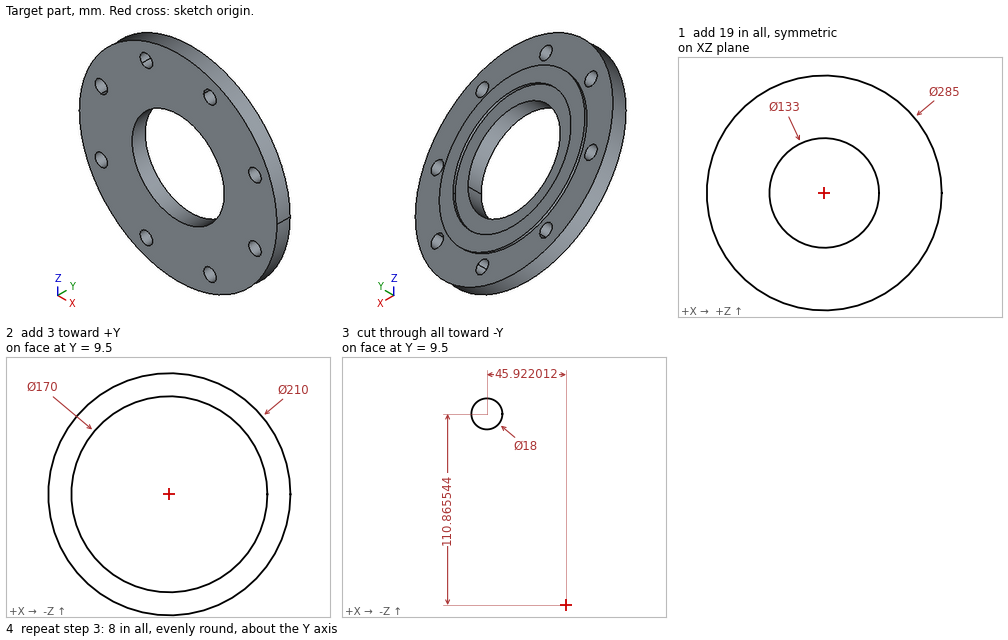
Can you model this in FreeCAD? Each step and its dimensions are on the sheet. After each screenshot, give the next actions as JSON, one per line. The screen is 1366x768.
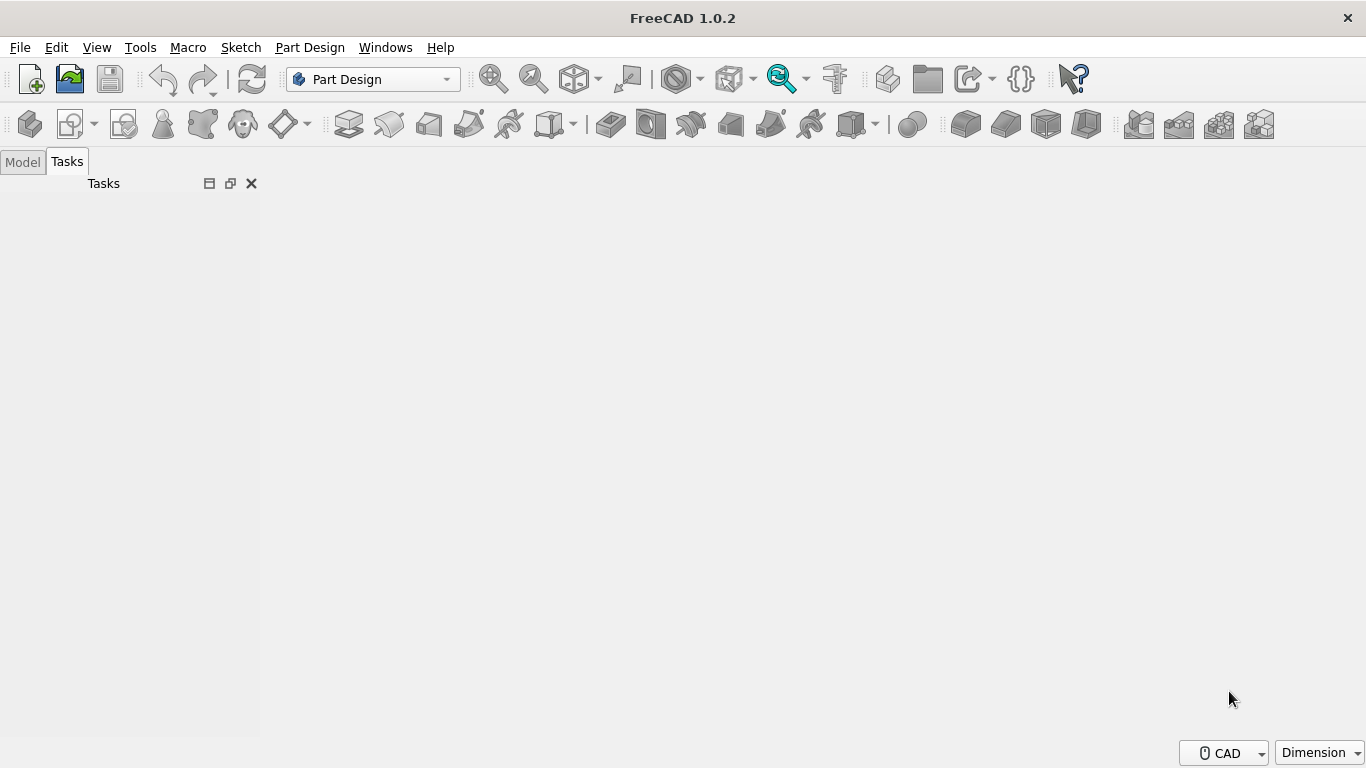
{"action": "key", "text": "ctrl+n"}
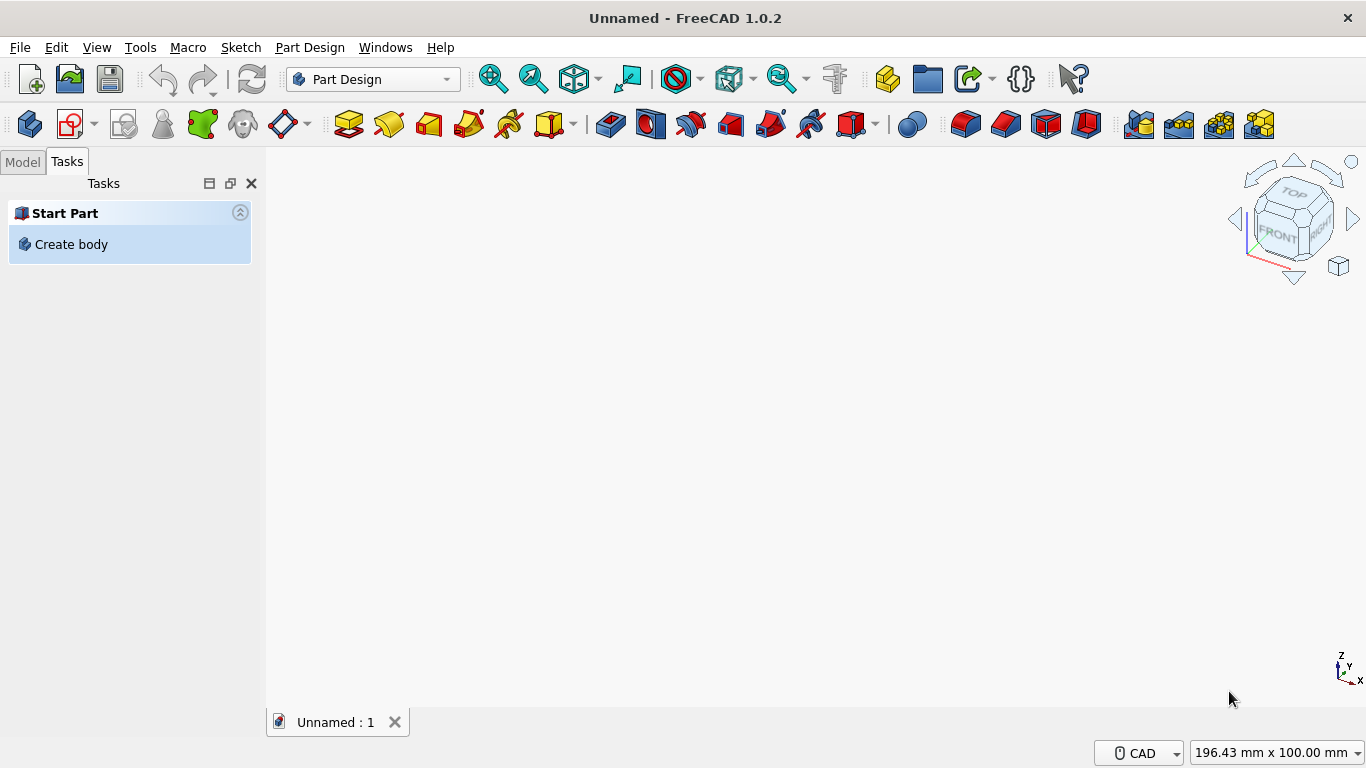
{"action": "left_click", "coordinate": [70, 124]}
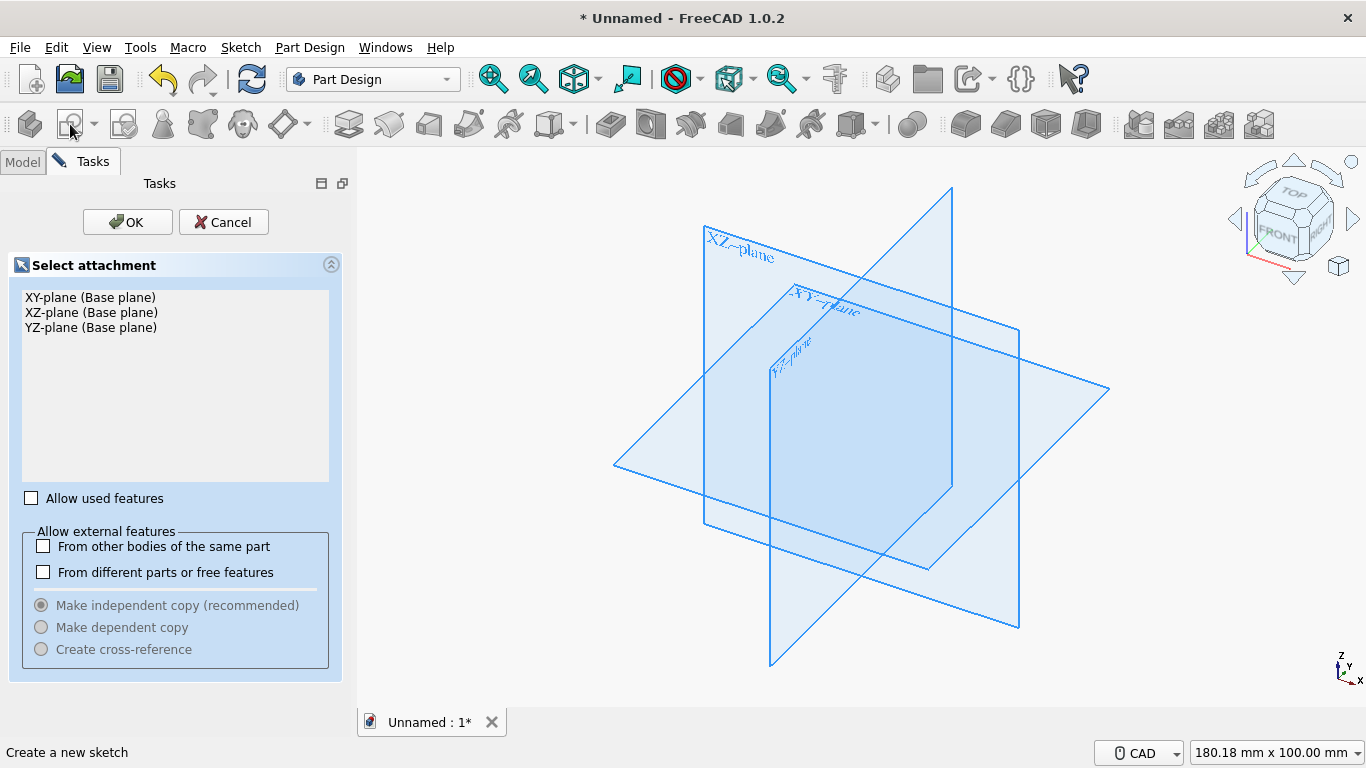
{"action": "left_click", "coordinate": [82, 312]}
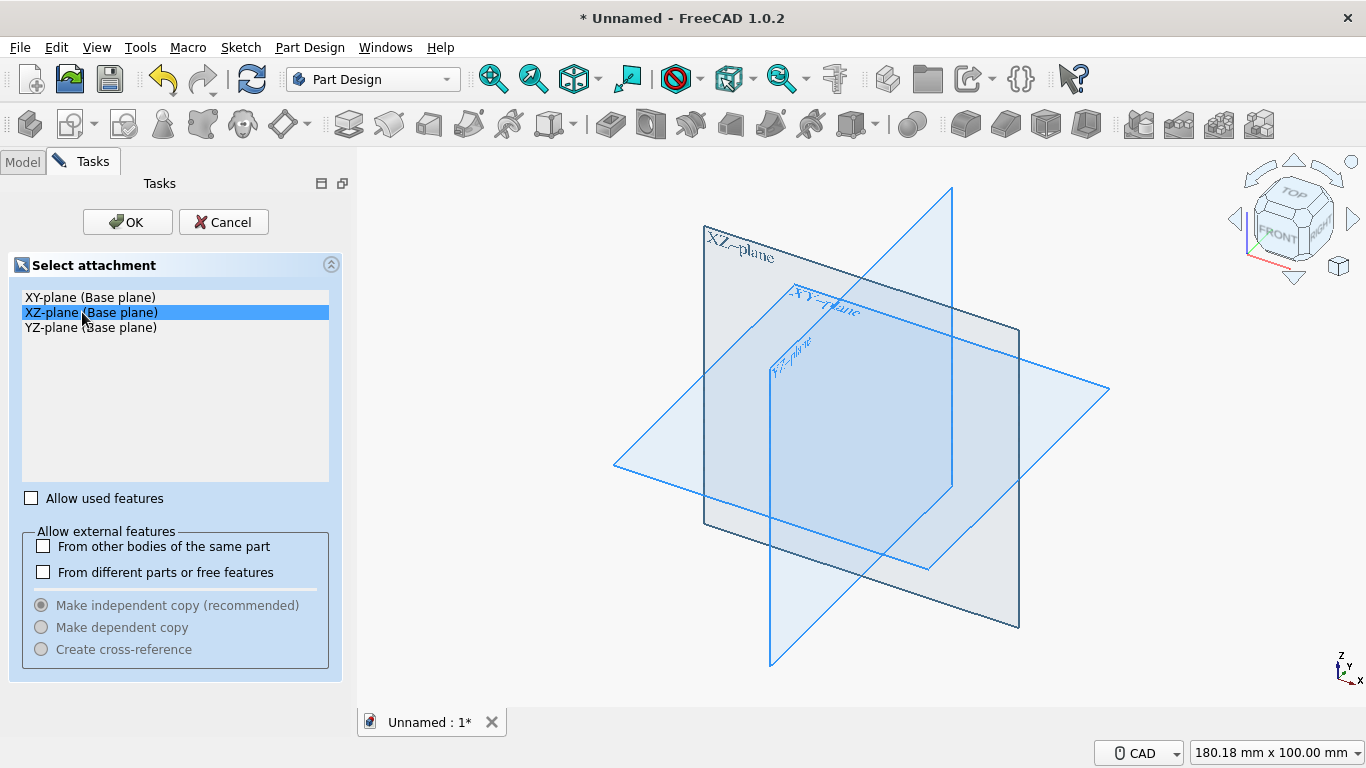
{"action": "left_click", "coordinate": [128, 222]}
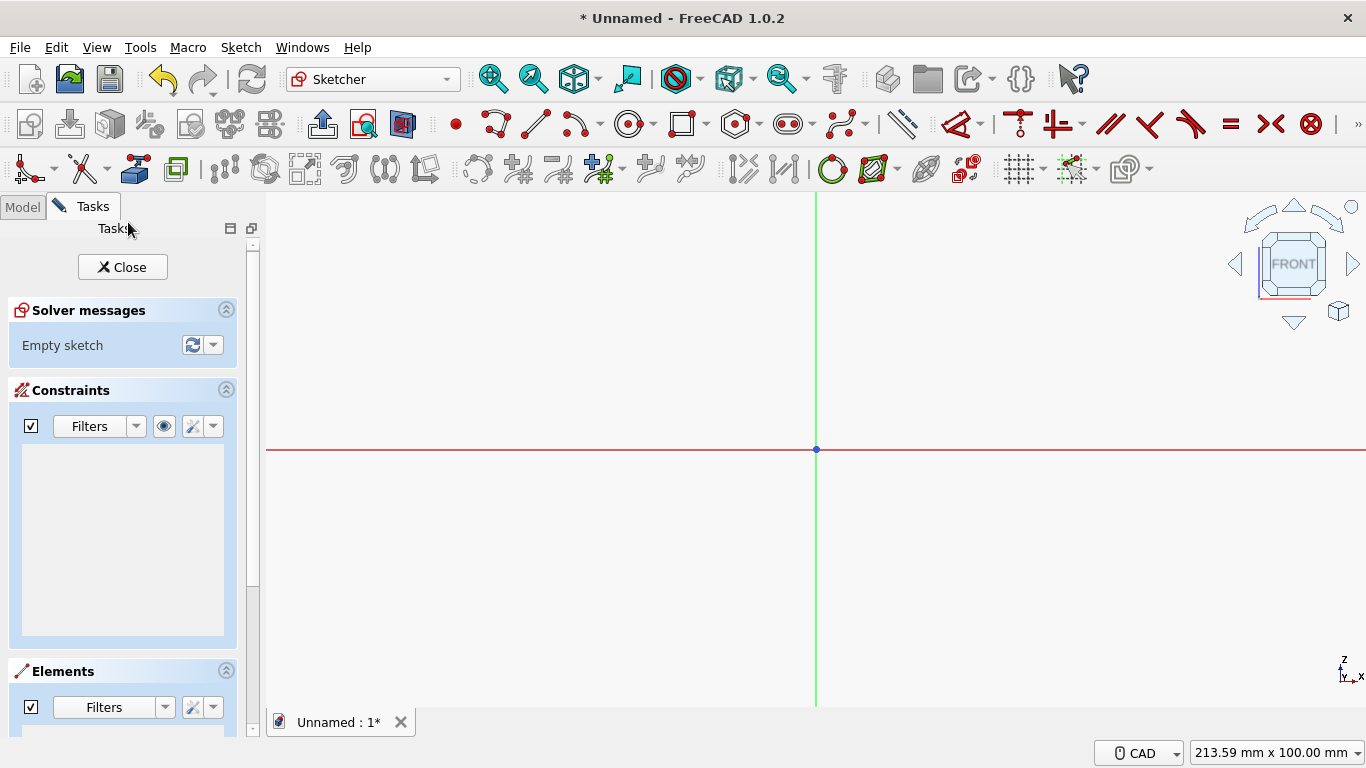
{"action": "scroll", "coordinate": [730, 449], "scroll_direction": "down", "scroll_amount": 8}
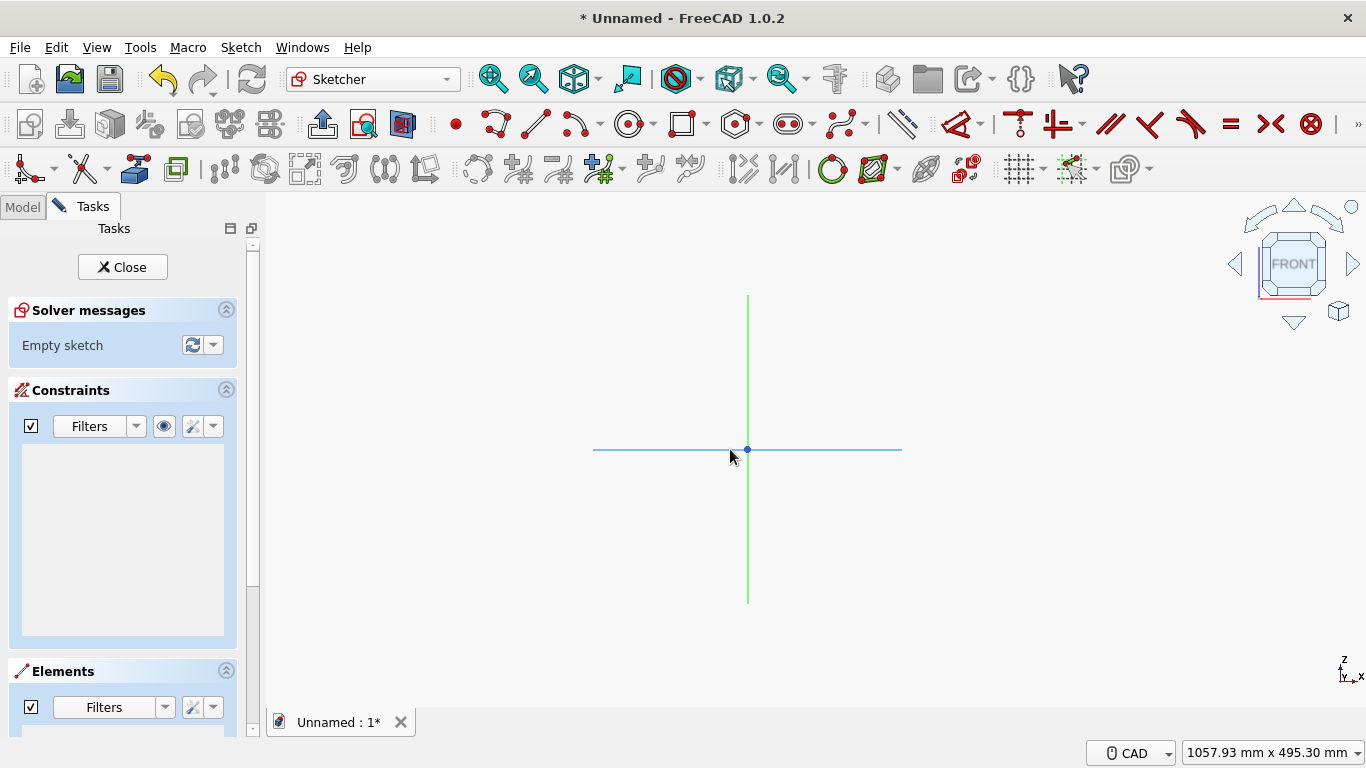
{"action": "key", "text": "g c"}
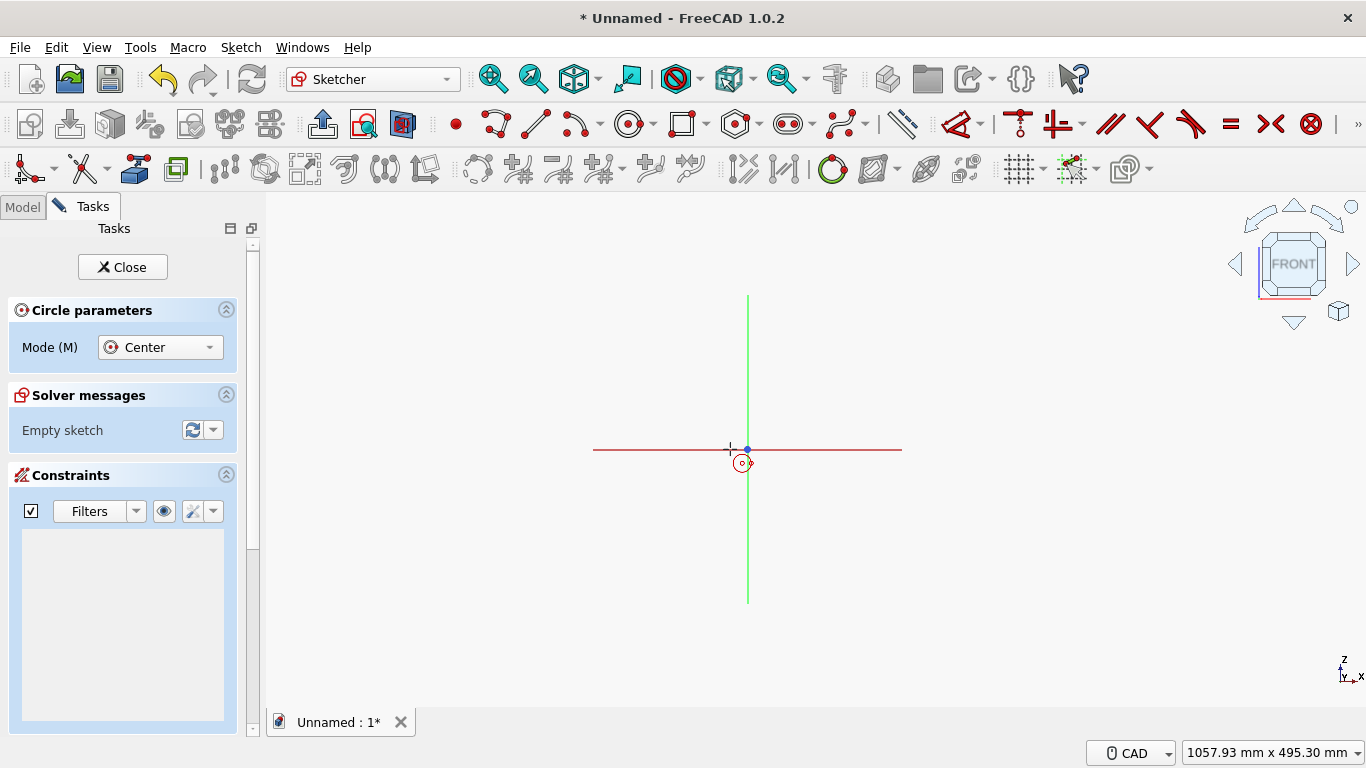
{"action": "left_click", "coordinate": [748, 450]}
{"action": "mouse_move", "coordinate": [852, 345]}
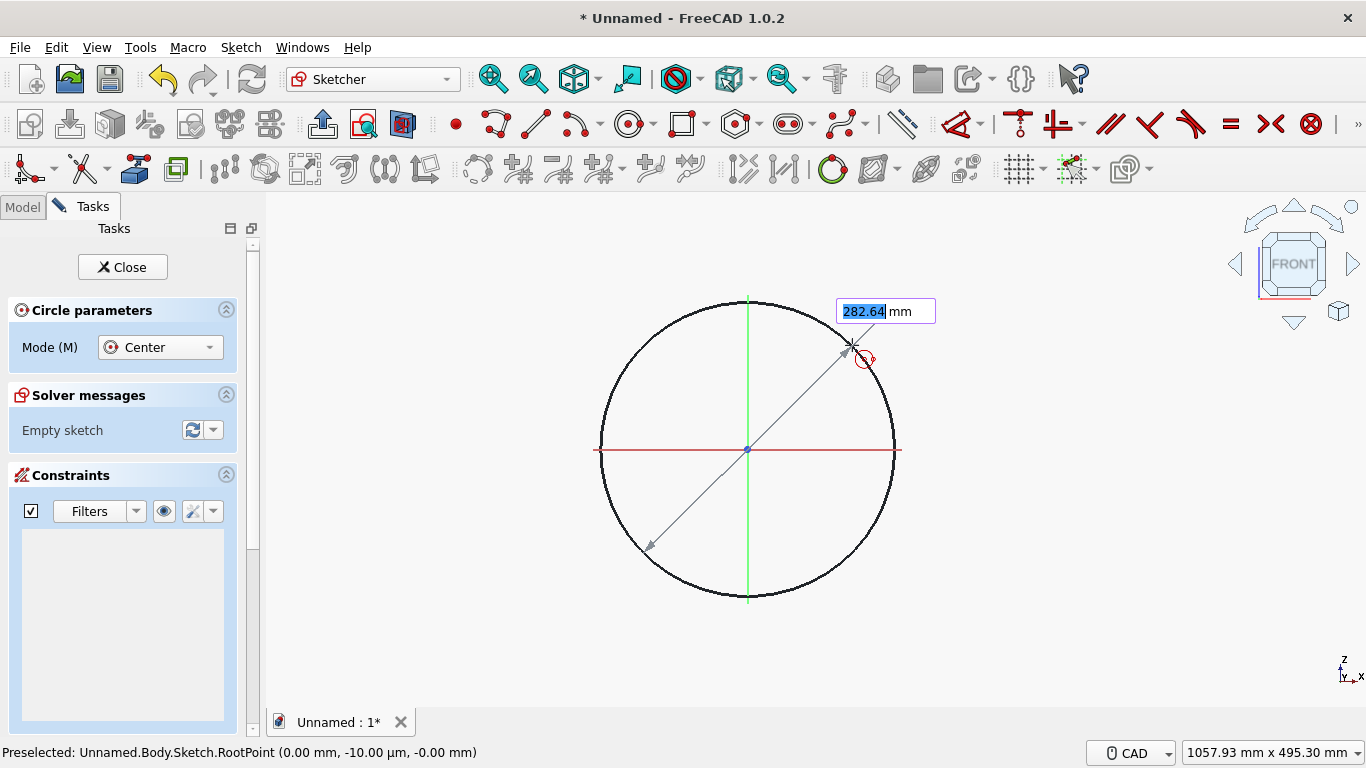
{"action": "type", "text": "285"}
{"action": "key", "text": "Return"}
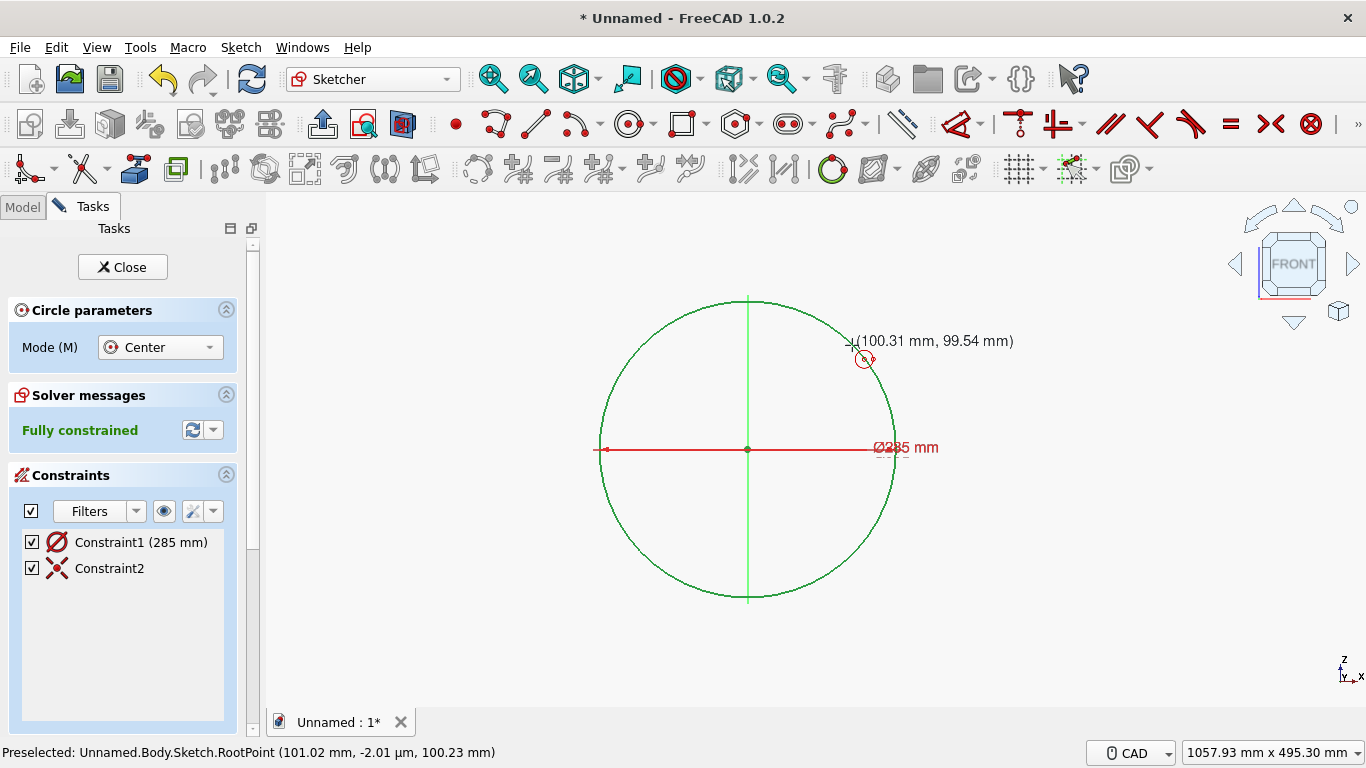
{"action": "left_click", "coordinate": [748, 450]}
{"action": "mouse_move", "coordinate": [797, 401]}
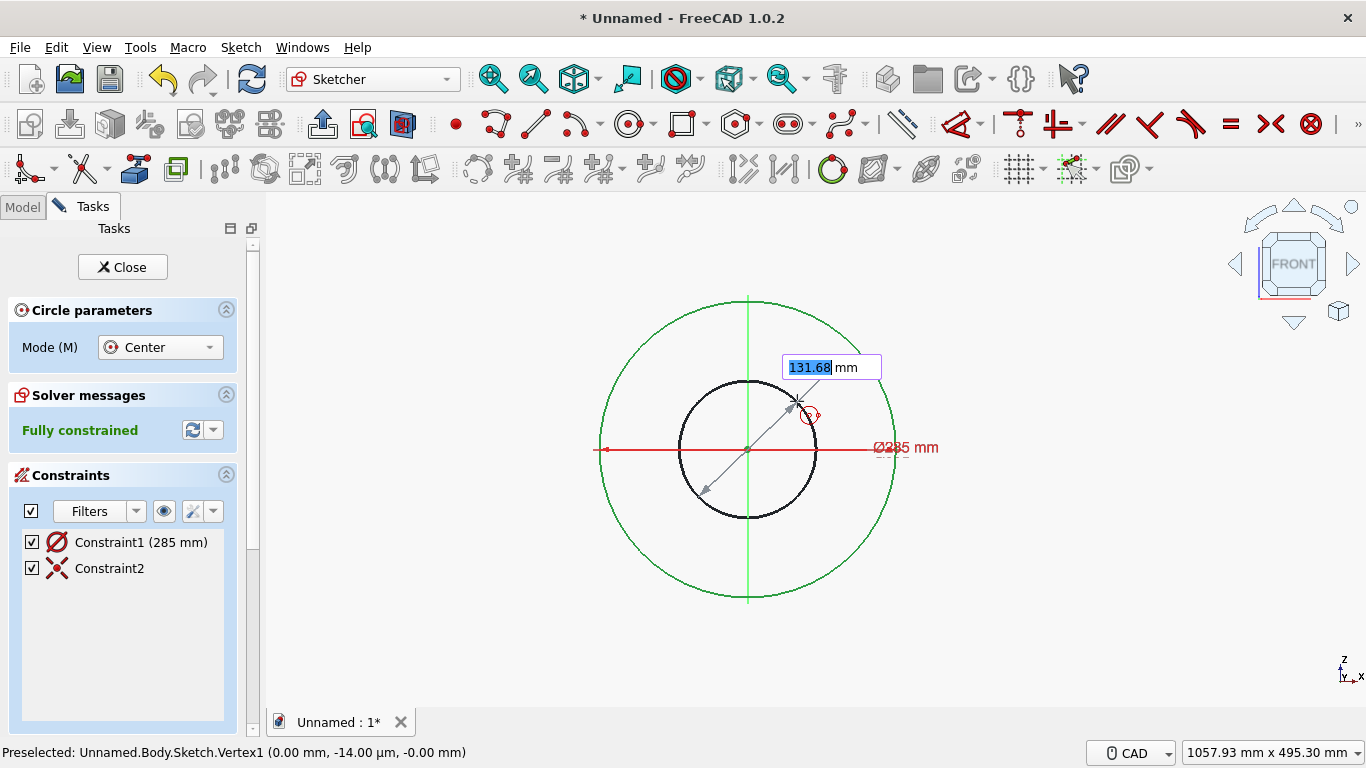
{"action": "type", "text": "133"}
{"action": "key", "text": "Return"}
{"action": "key", "text": "Escape"}